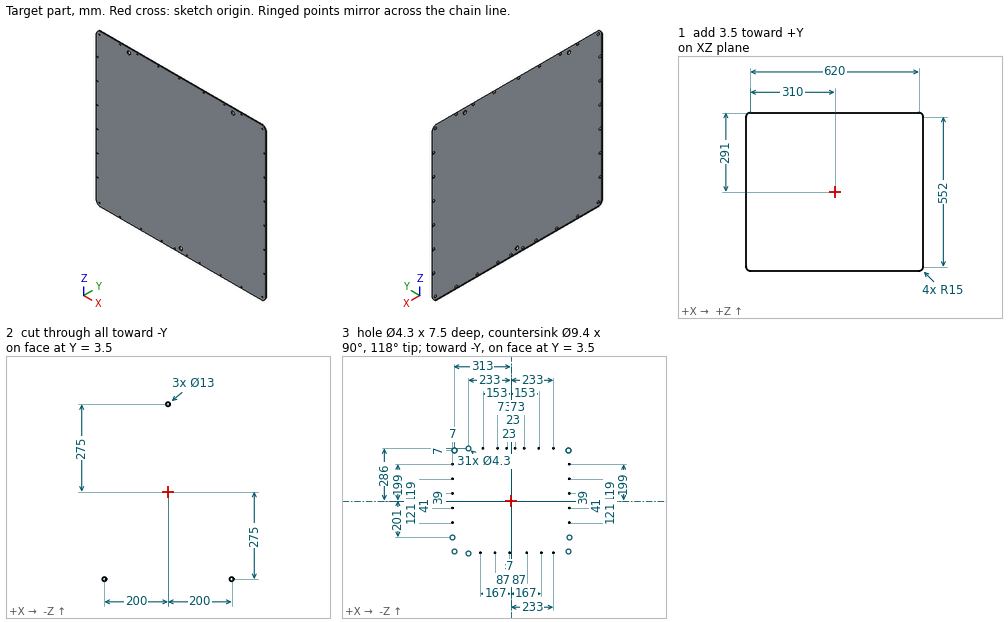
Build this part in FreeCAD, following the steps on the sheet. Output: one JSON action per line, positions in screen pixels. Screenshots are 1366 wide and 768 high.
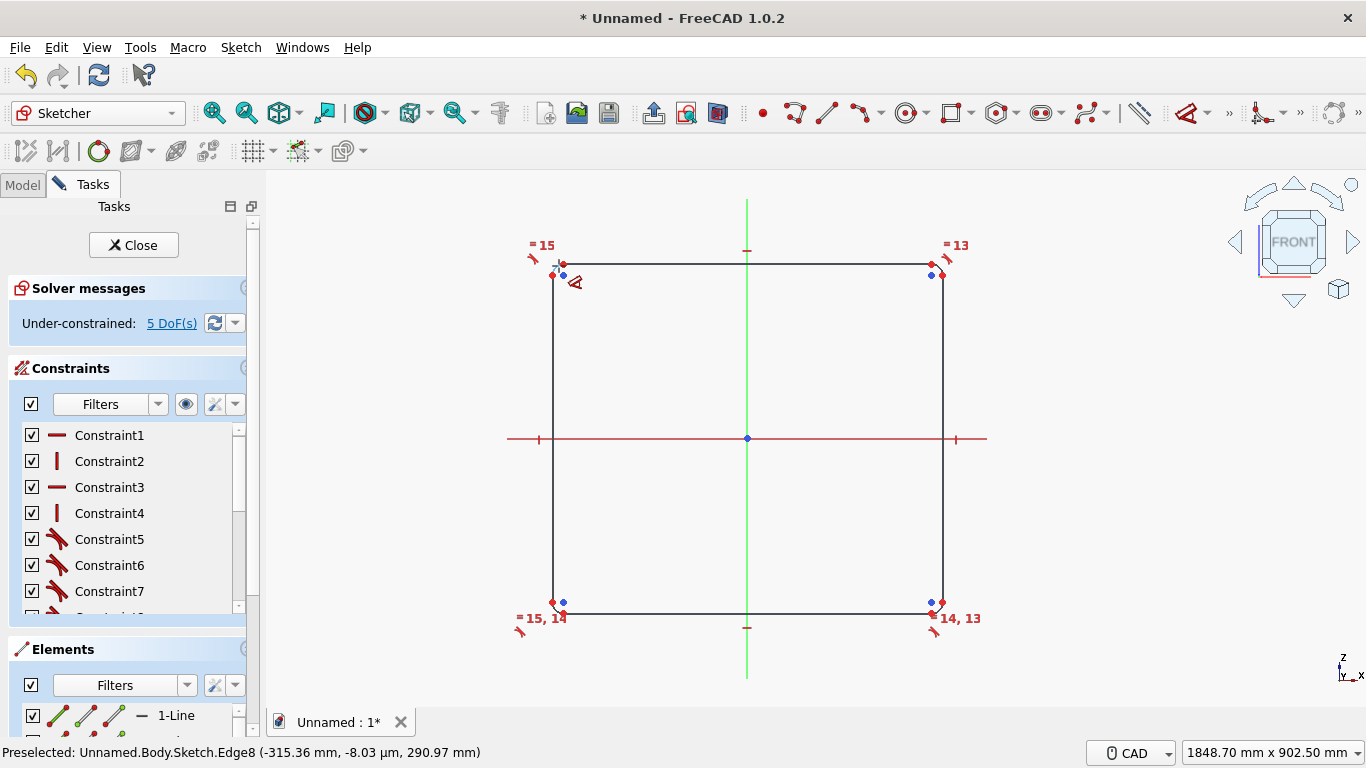
{"action": "scroll", "coordinate": [942, 270], "scroll_direction": "up", "scroll_amount": 8}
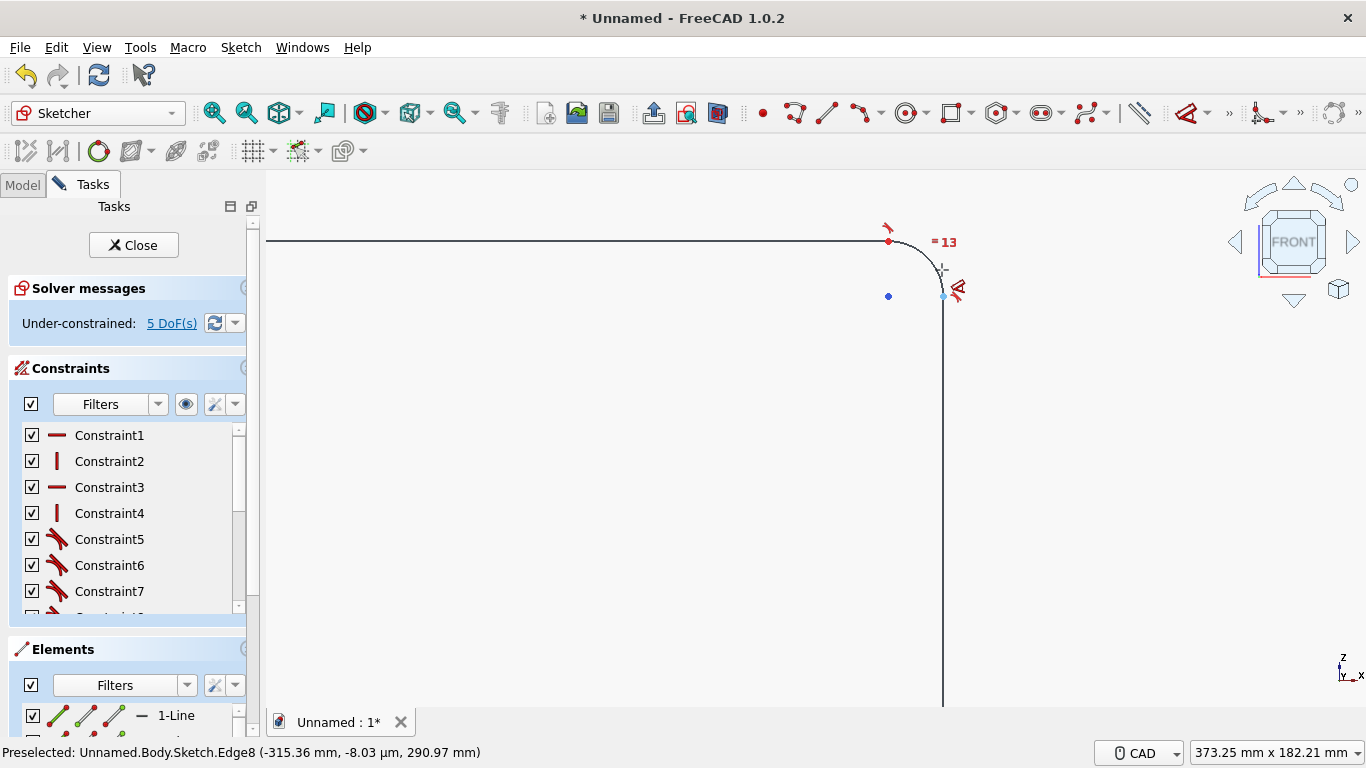
{"action": "left_click", "coordinate": [937, 271]}
{"action": "left_click", "coordinate": [965, 256]}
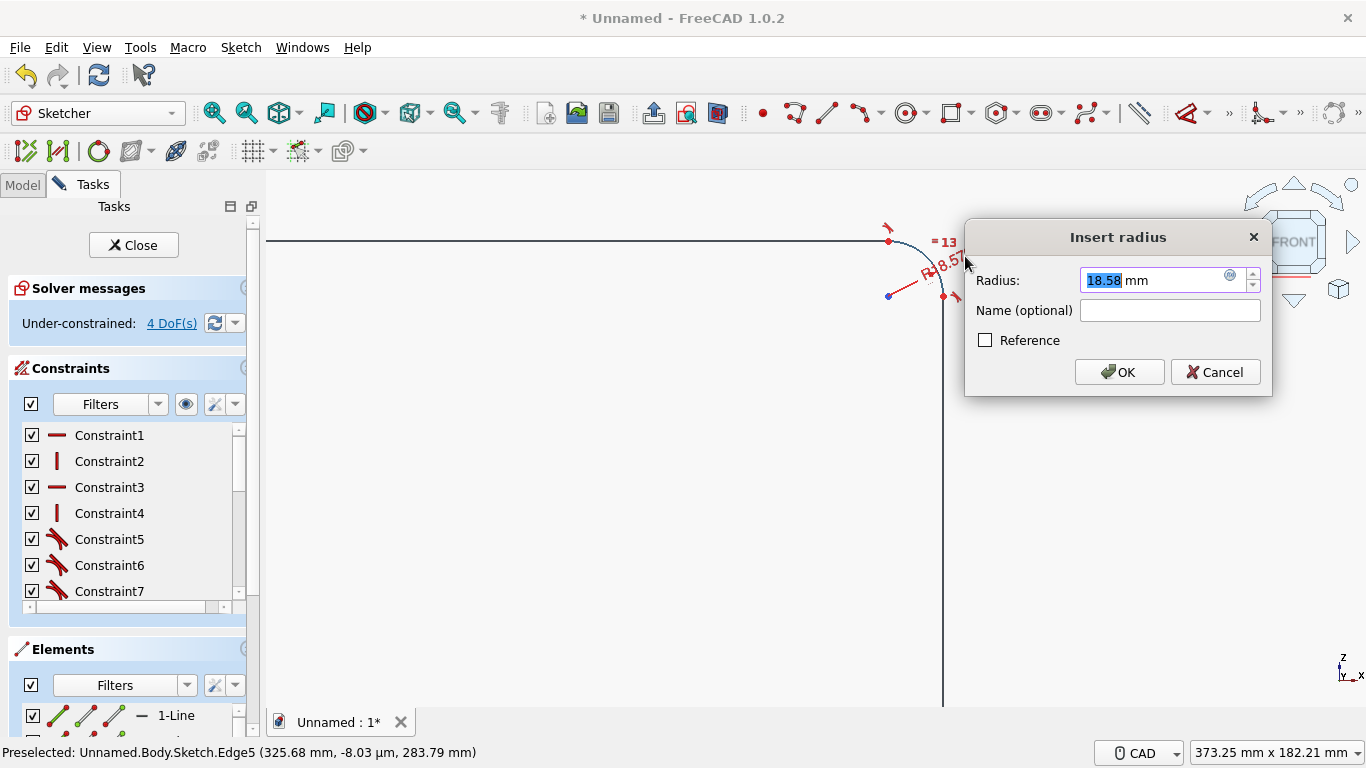
{"action": "type", "text": "15"}
{"action": "key", "text": "Return"}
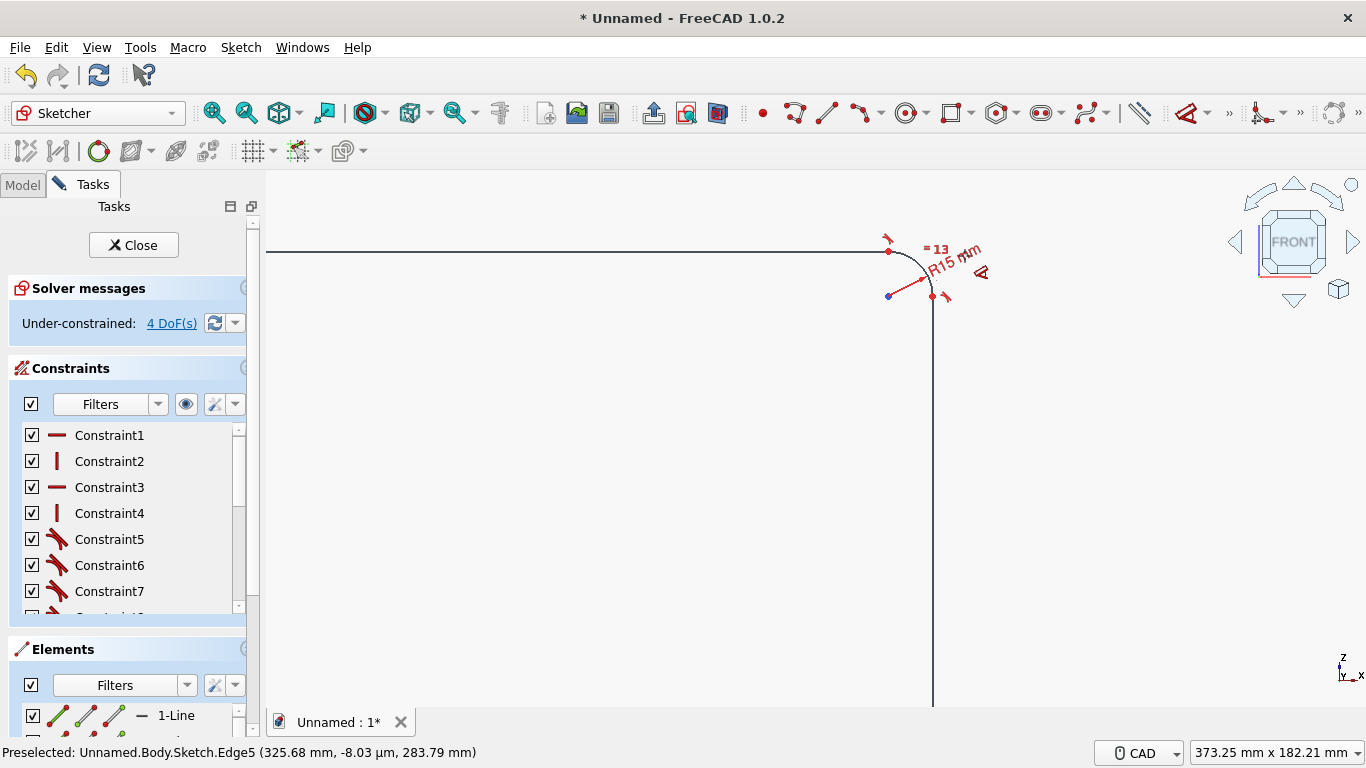
{"action": "scroll", "coordinate": [943, 270], "scroll_direction": "down", "scroll_amount": 8}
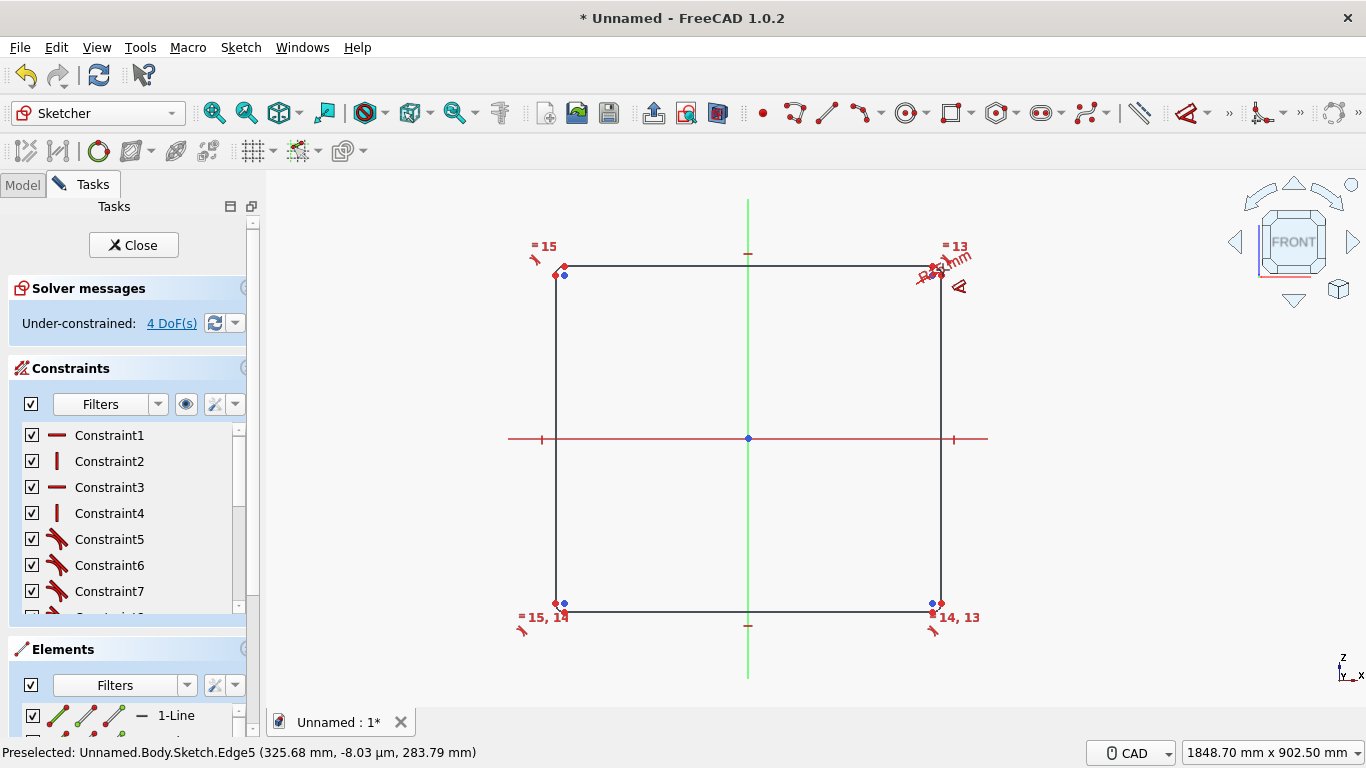
{"action": "left_click", "coordinate": [822, 266]}
{"action": "left_click", "coordinate": [664, 232]}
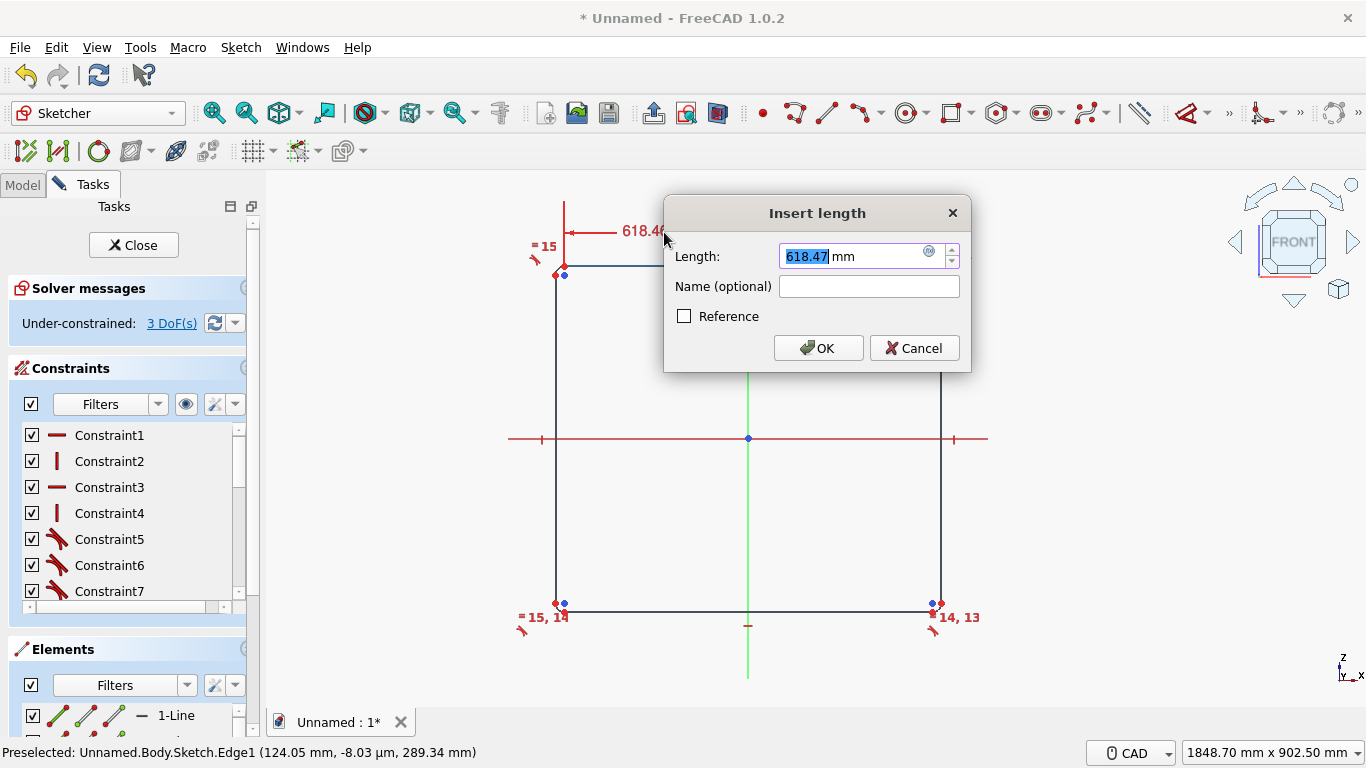
{"action": "type", "text": "620"}
{"action": "key", "text": "Return"}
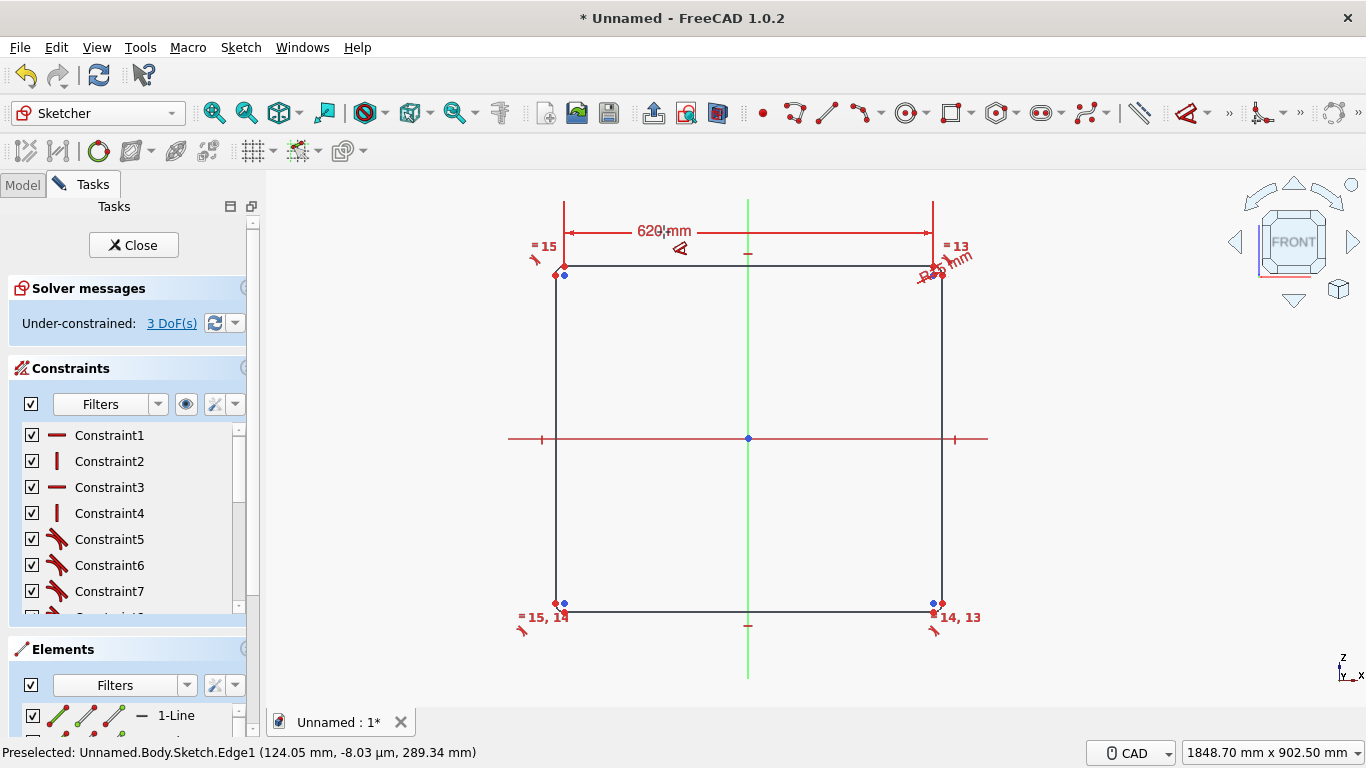
{"action": "left_click", "coordinate": [942, 374]}
{"action": "left_click", "coordinate": [976, 364]}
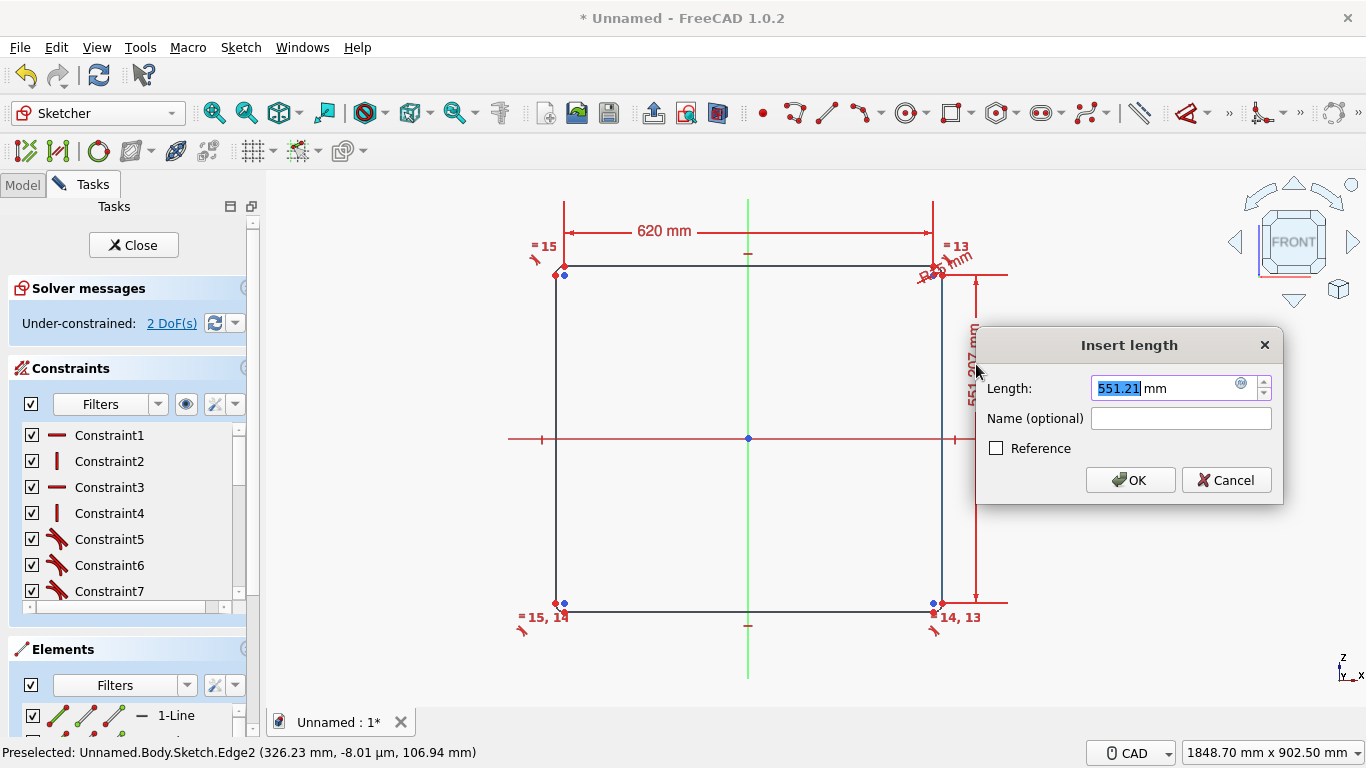
{"action": "type", "text": "552"}
{"action": "key", "text": "Return"}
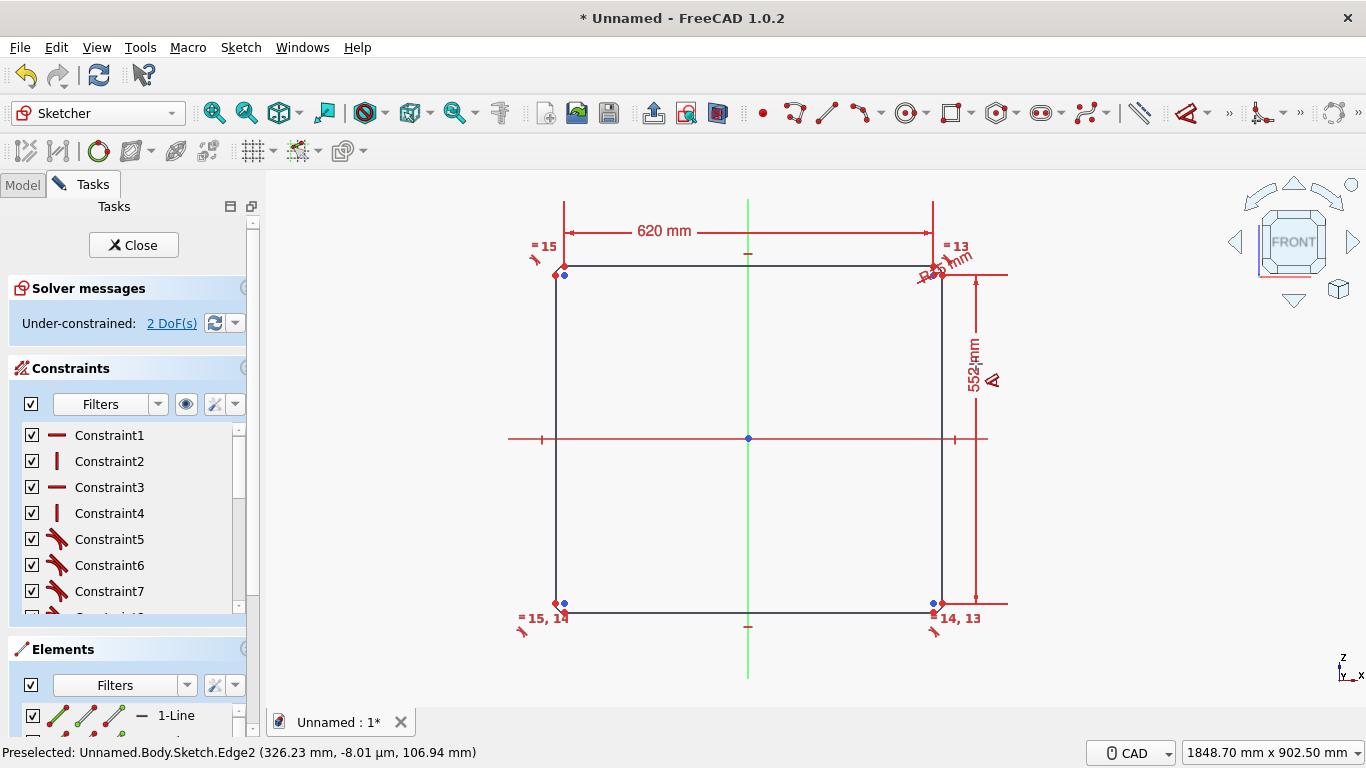
{"action": "scroll", "coordinate": [564, 266], "scroll_direction": "up", "scroll_amount": 2}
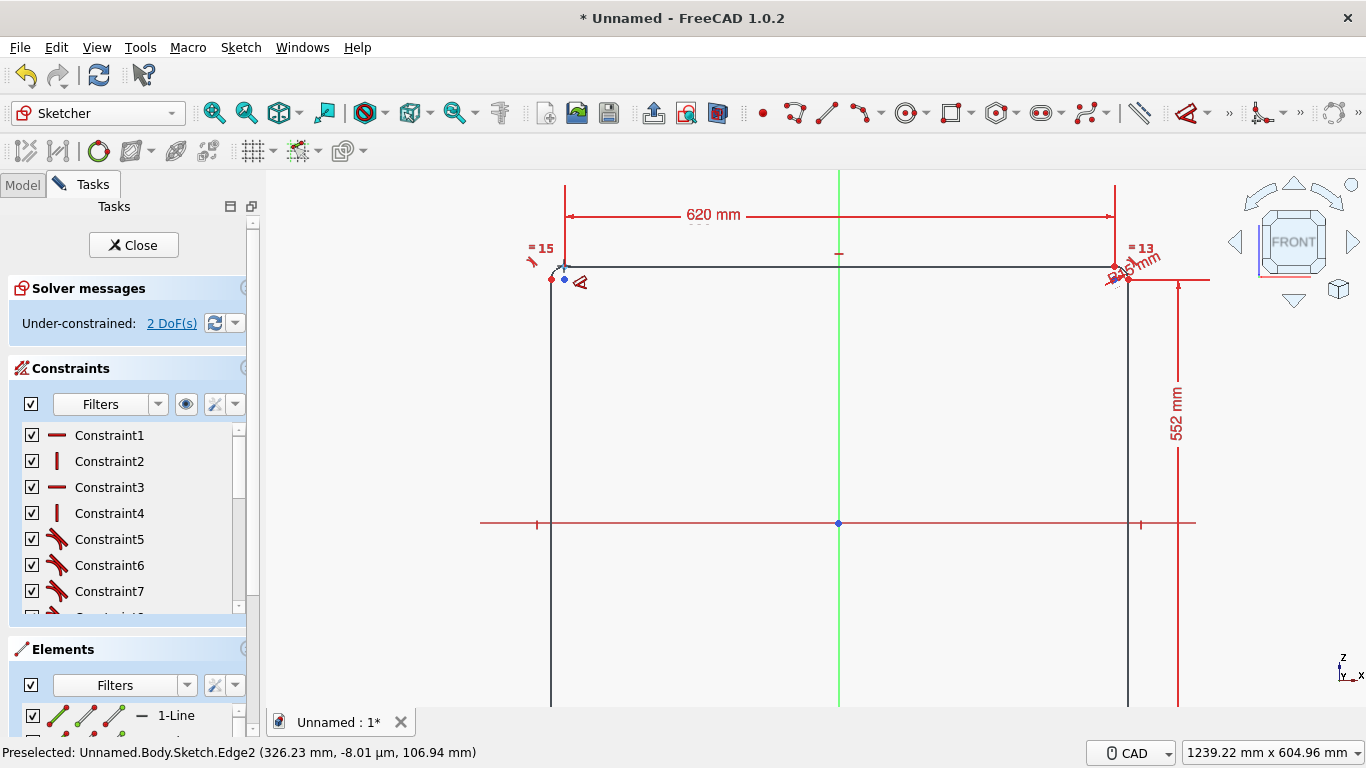
{"action": "left_click", "coordinate": [565, 267]}
{"action": "left_click", "coordinate": [639, 233]}